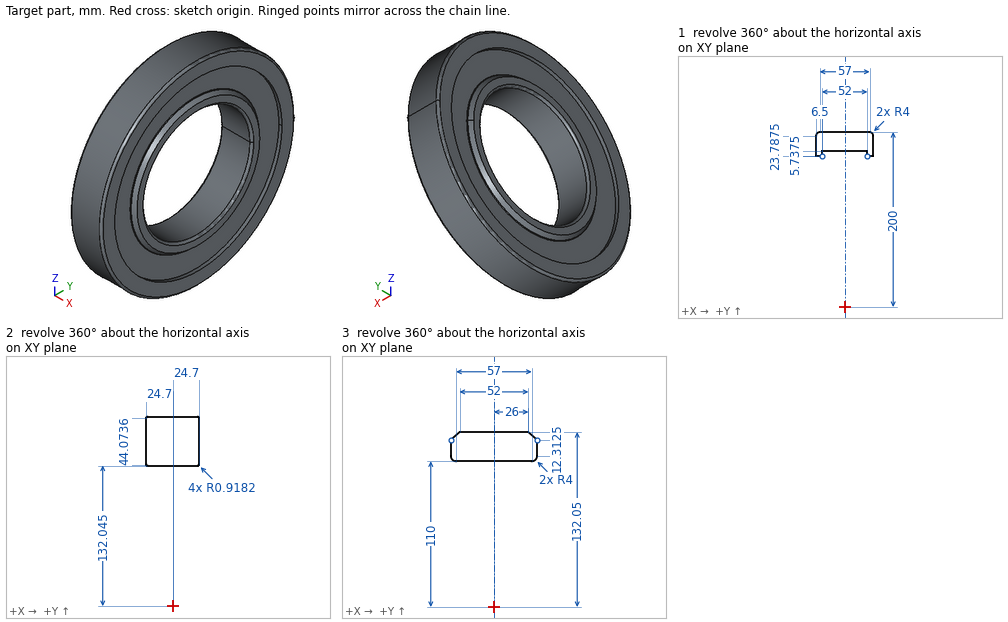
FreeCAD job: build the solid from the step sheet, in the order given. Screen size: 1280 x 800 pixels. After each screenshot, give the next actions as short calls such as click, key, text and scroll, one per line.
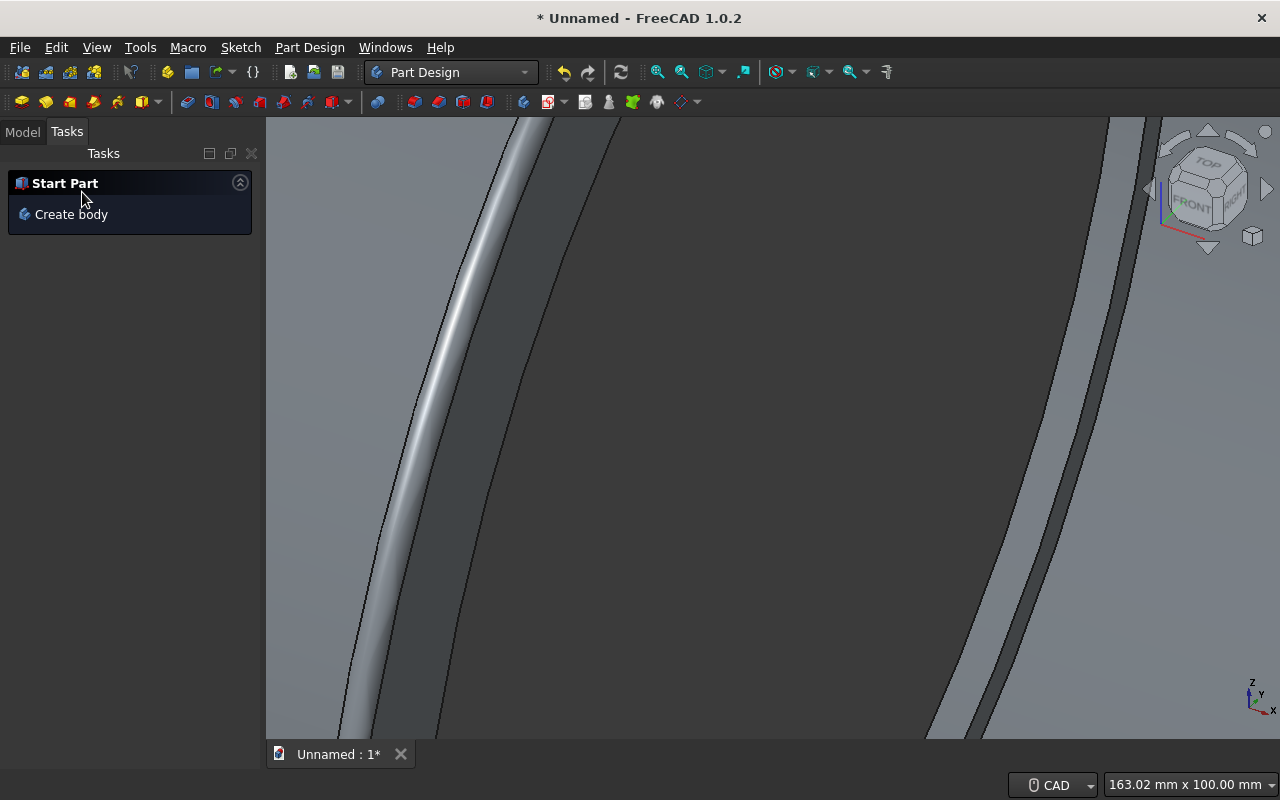
click(658, 72)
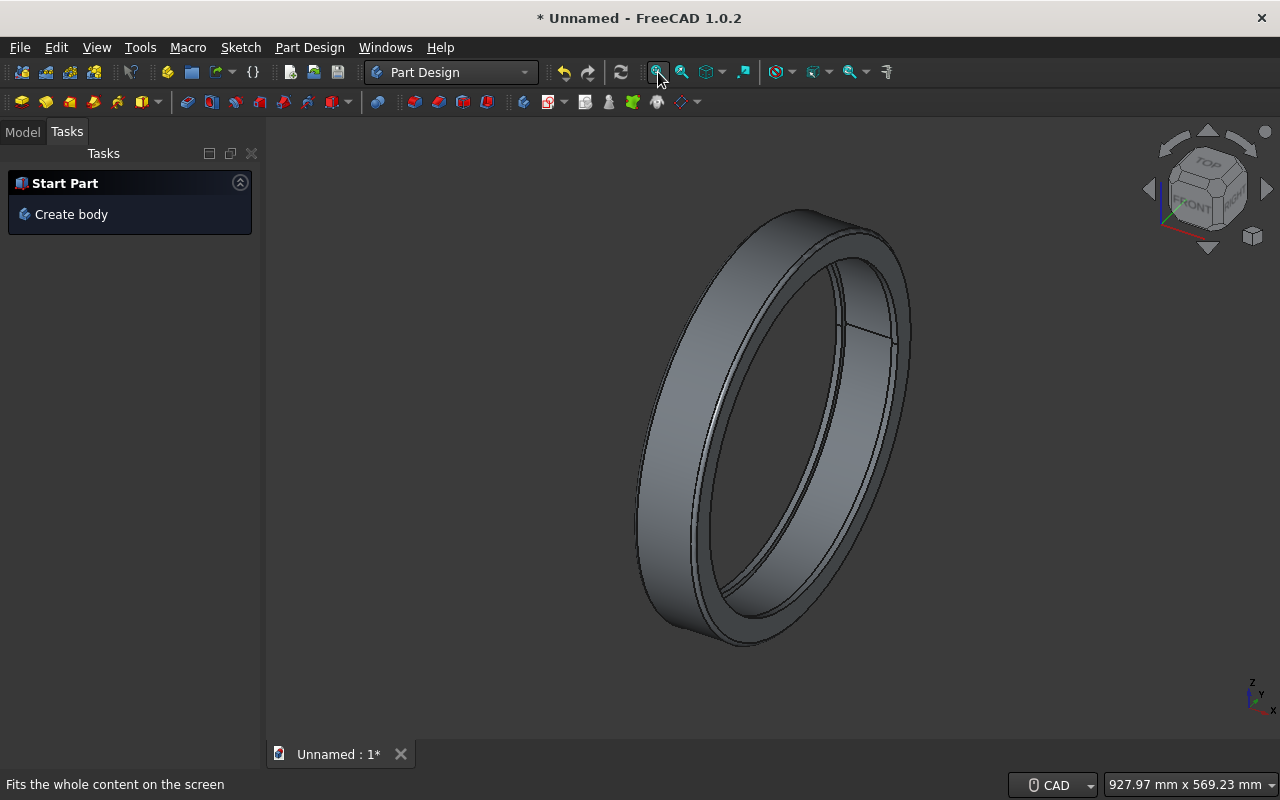
click(548, 102)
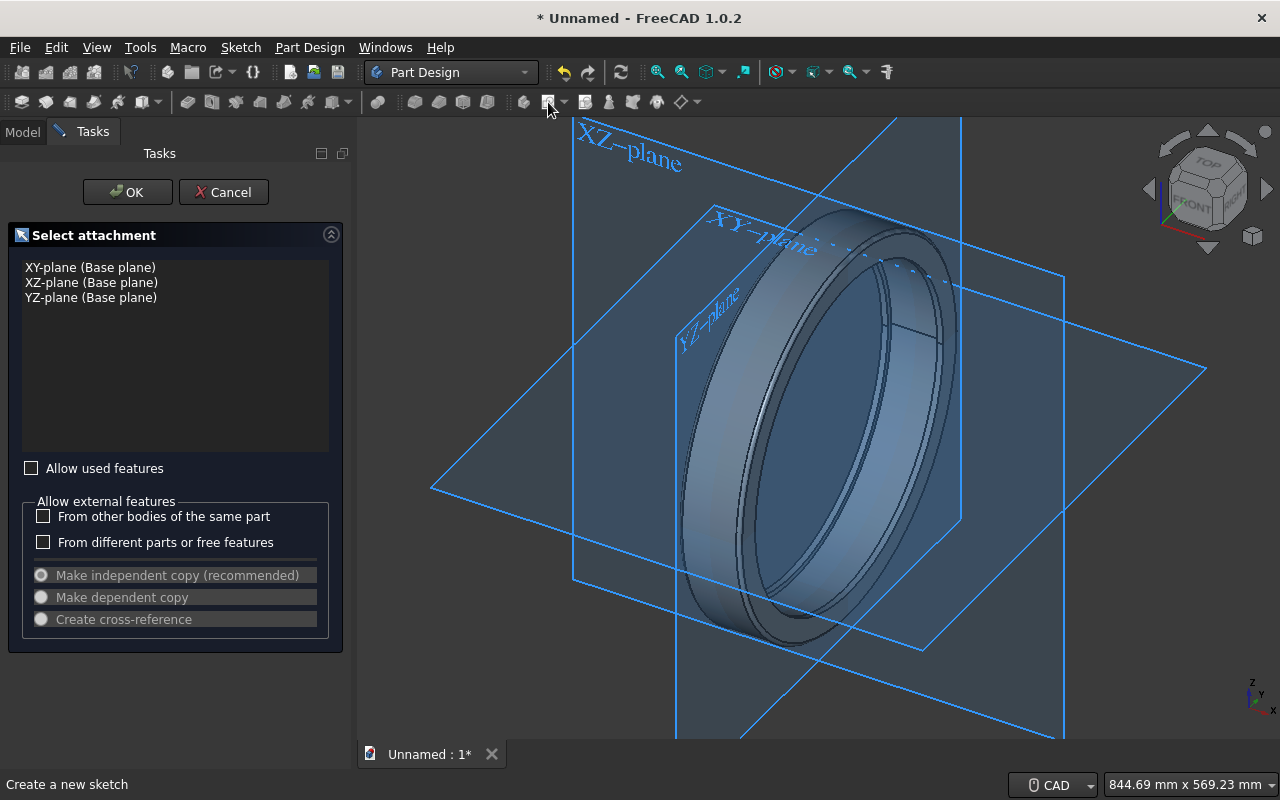
click(82, 268)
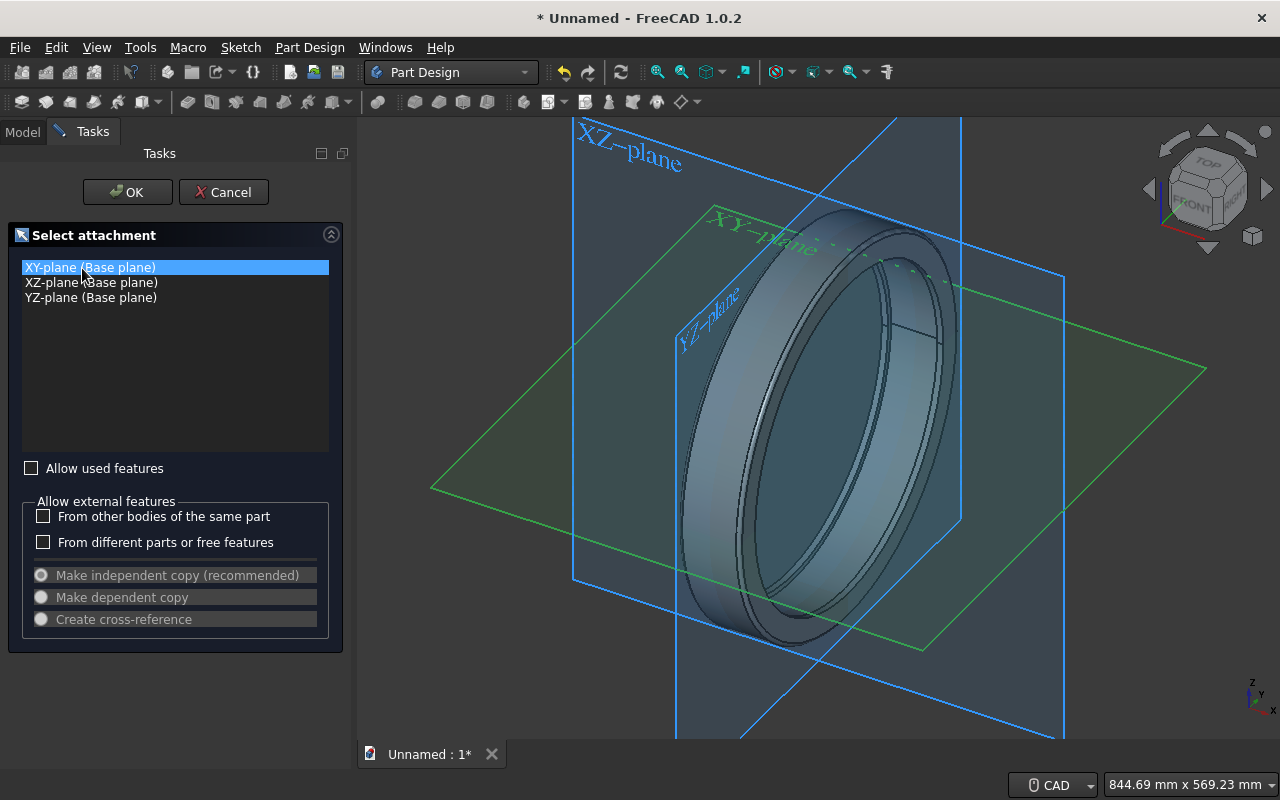
click(128, 192)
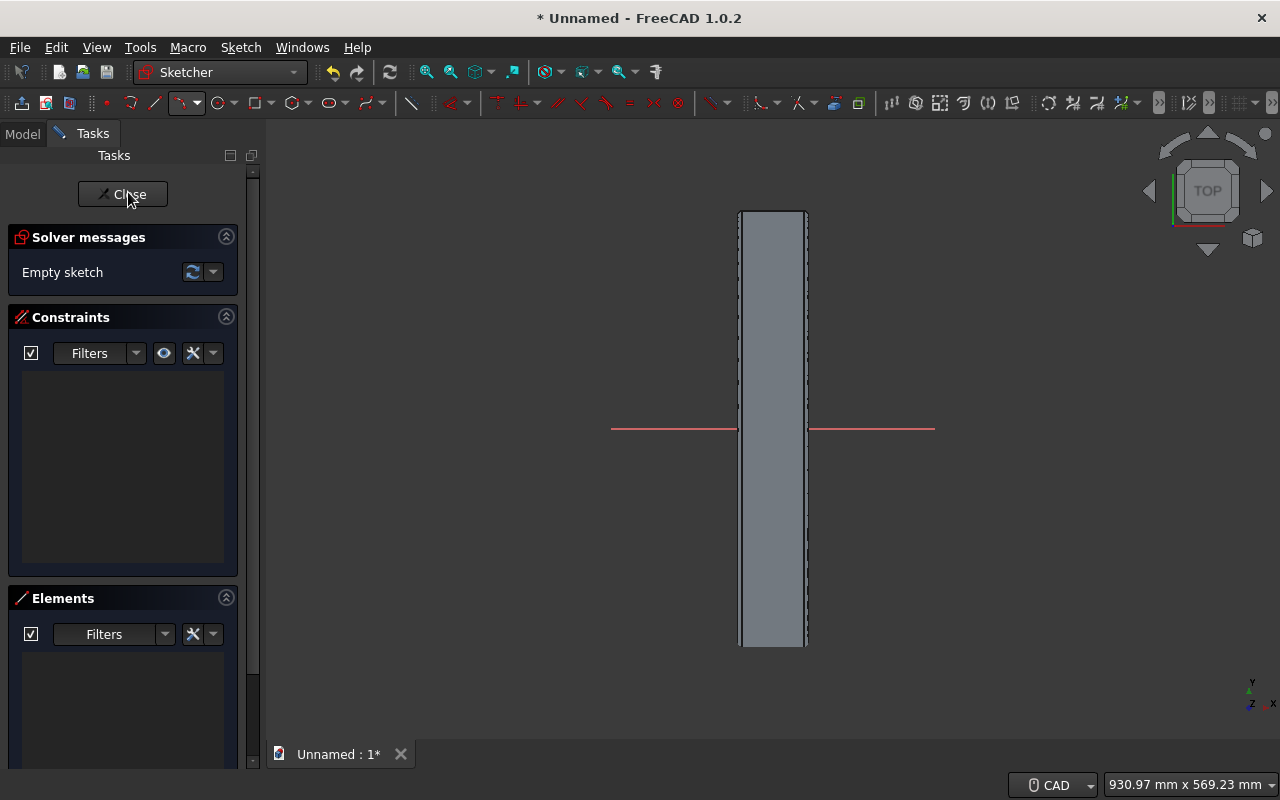
click(70, 104)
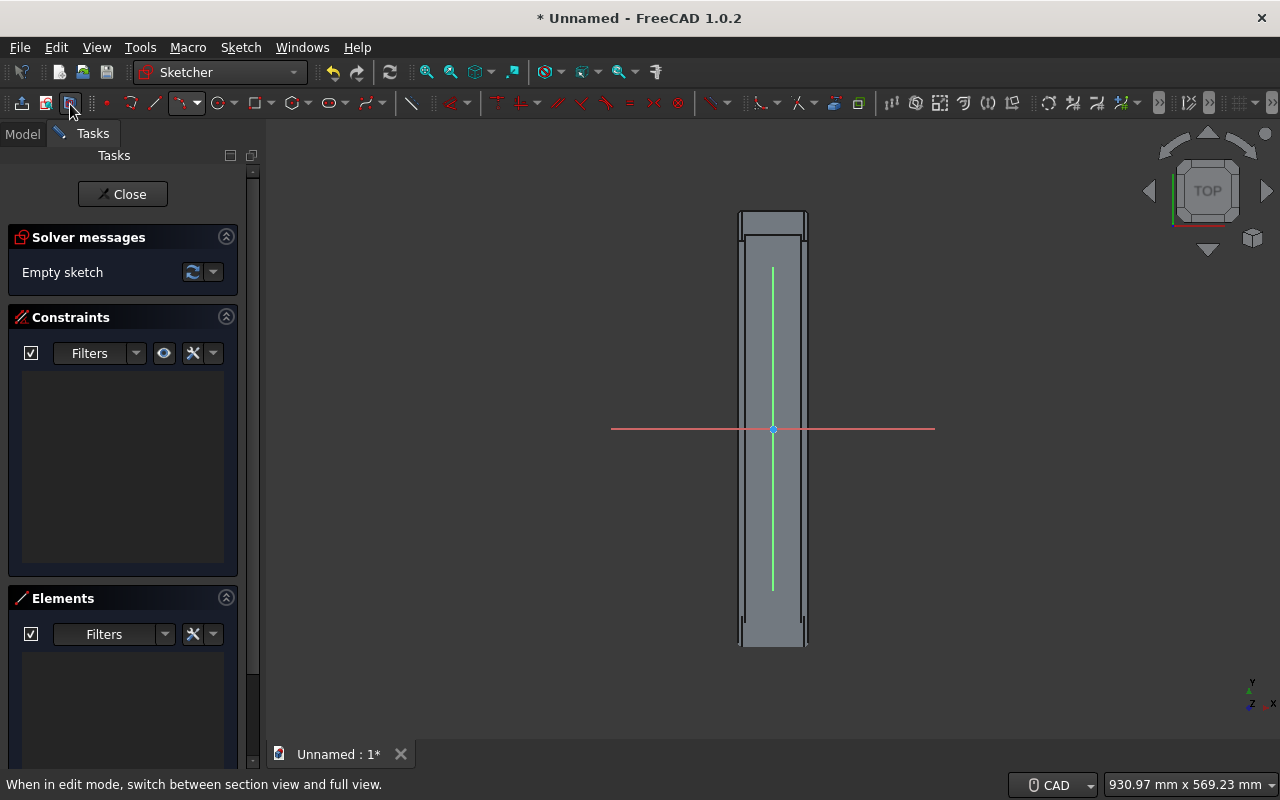
scroll(784, 234, up, 10)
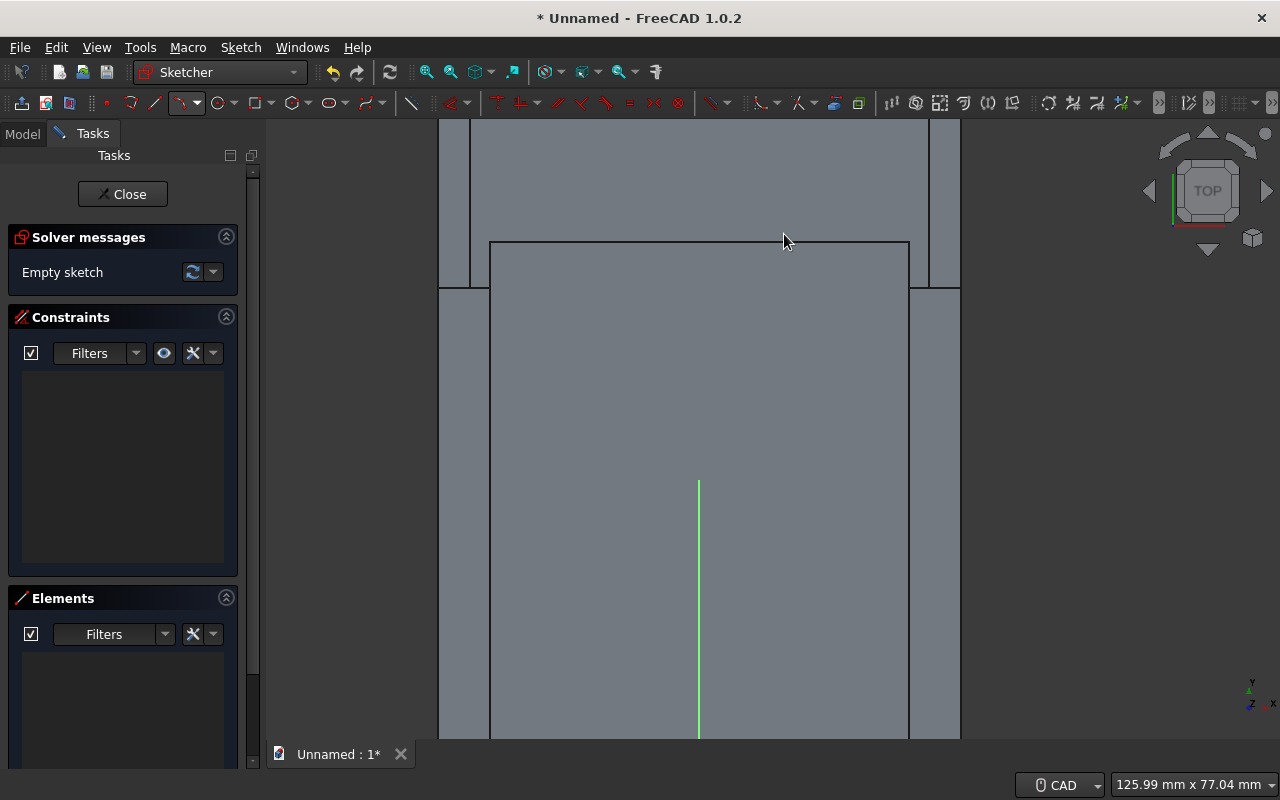
click(156, 104)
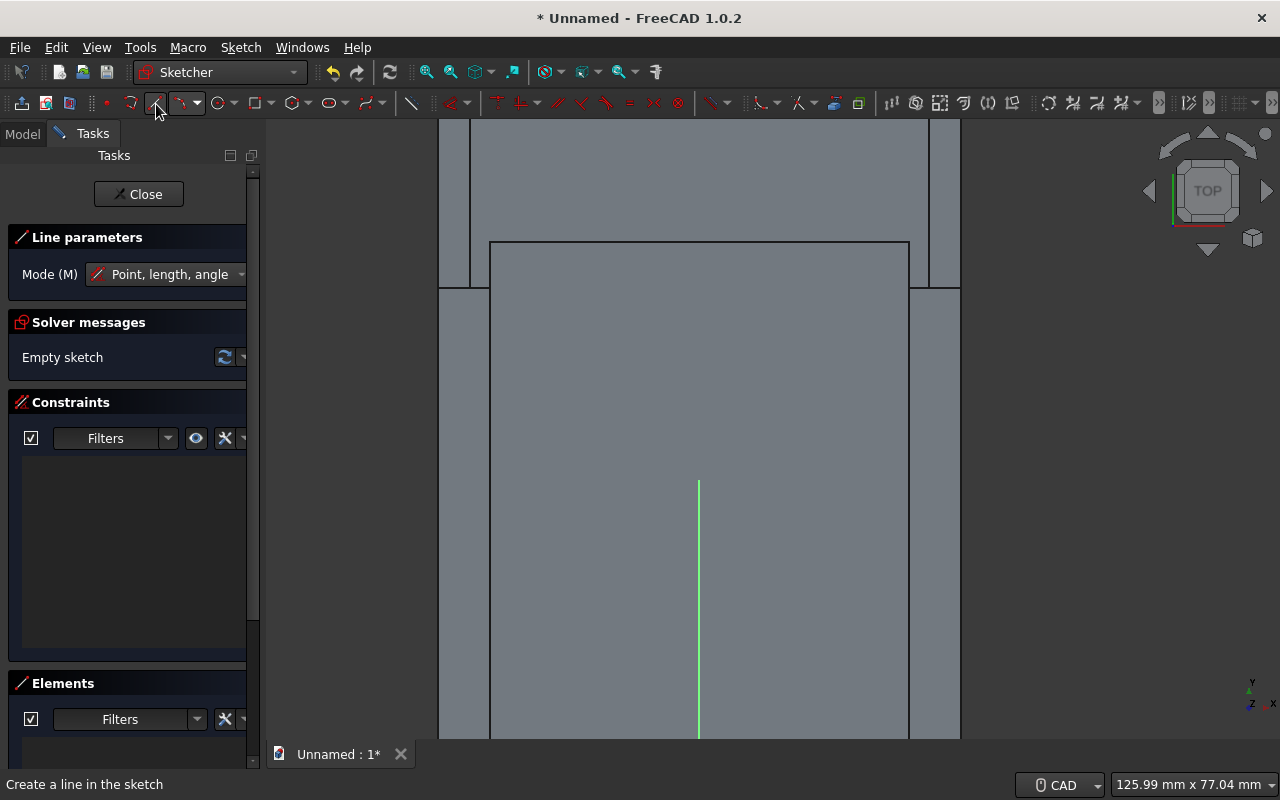
click(501, 249)
click(501, 604)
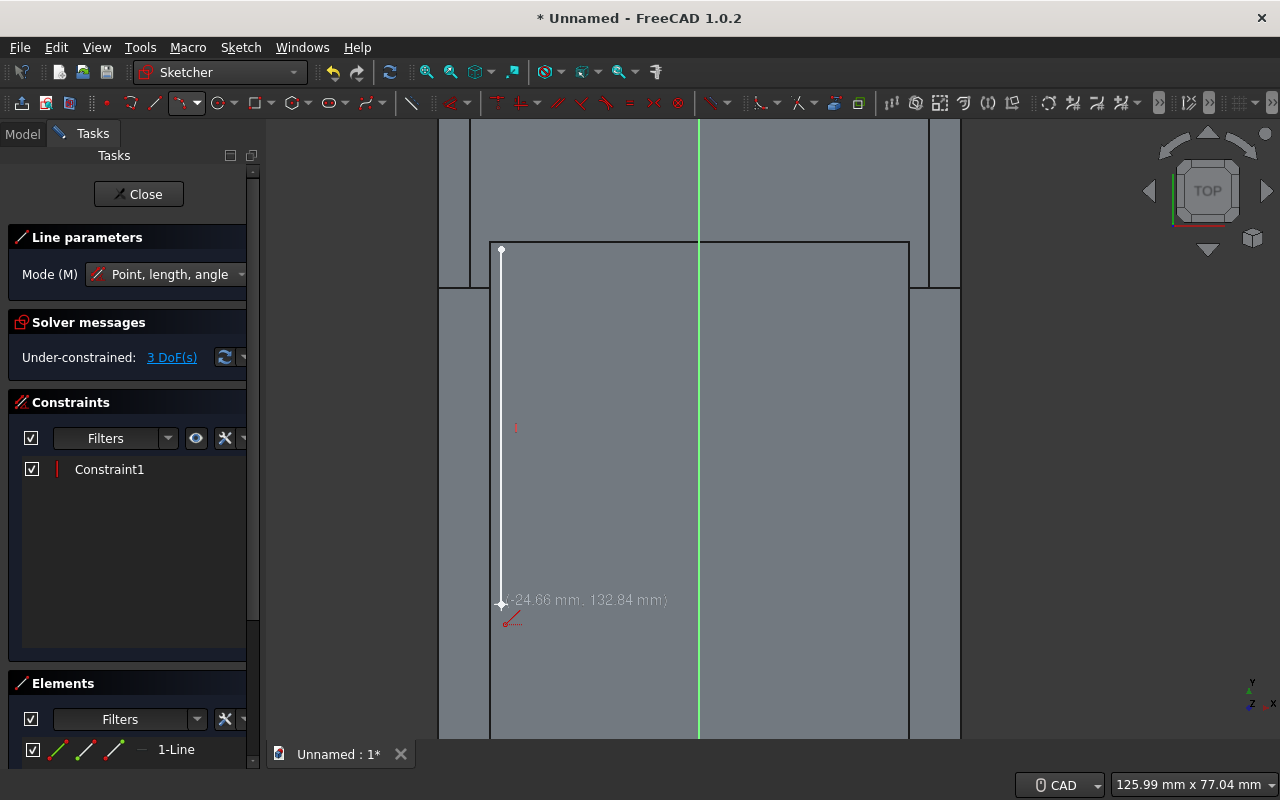
scroll(508, 611, up, 3)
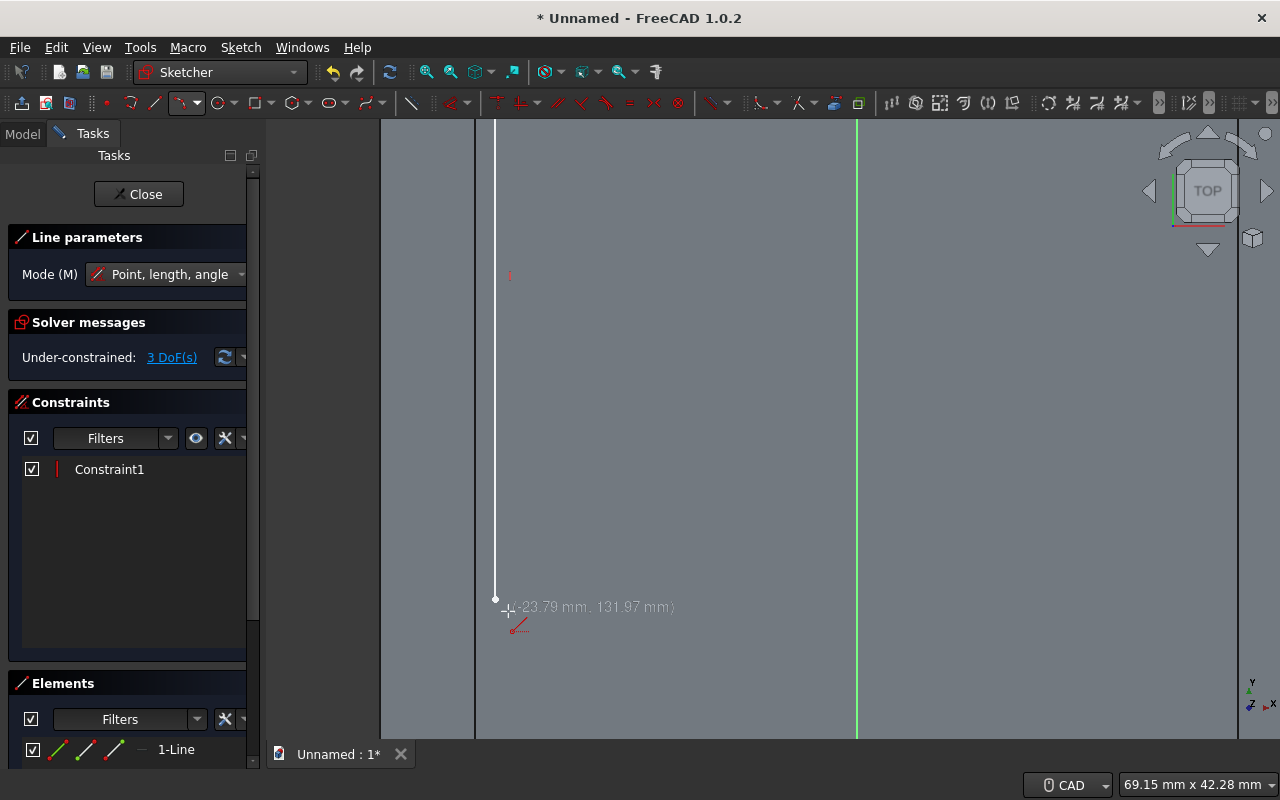
click(508, 611)